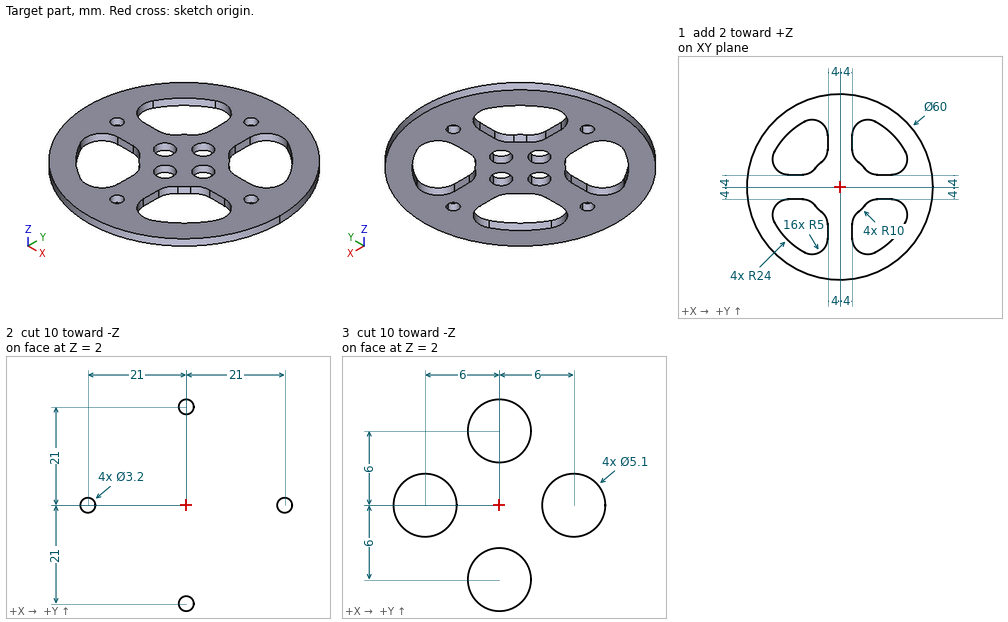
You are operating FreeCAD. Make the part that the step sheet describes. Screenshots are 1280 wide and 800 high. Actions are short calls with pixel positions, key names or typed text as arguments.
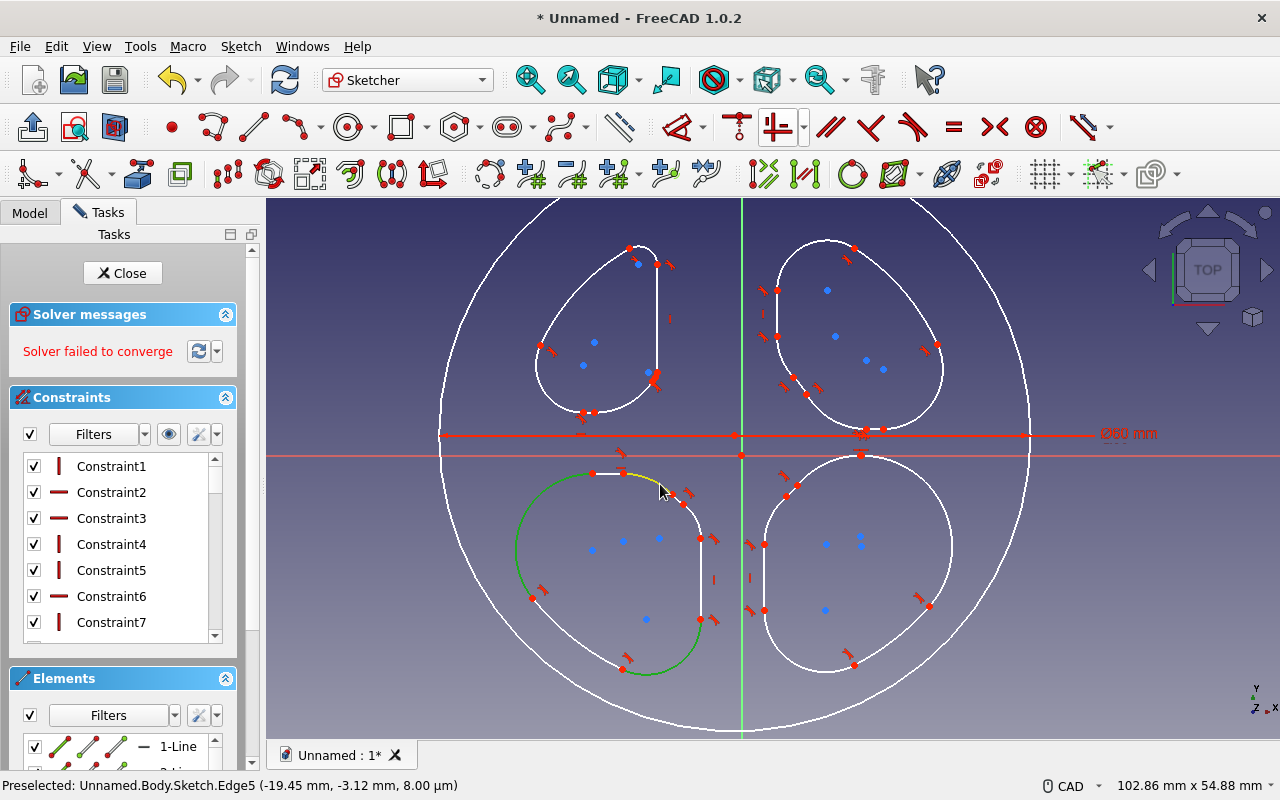
click(660, 484)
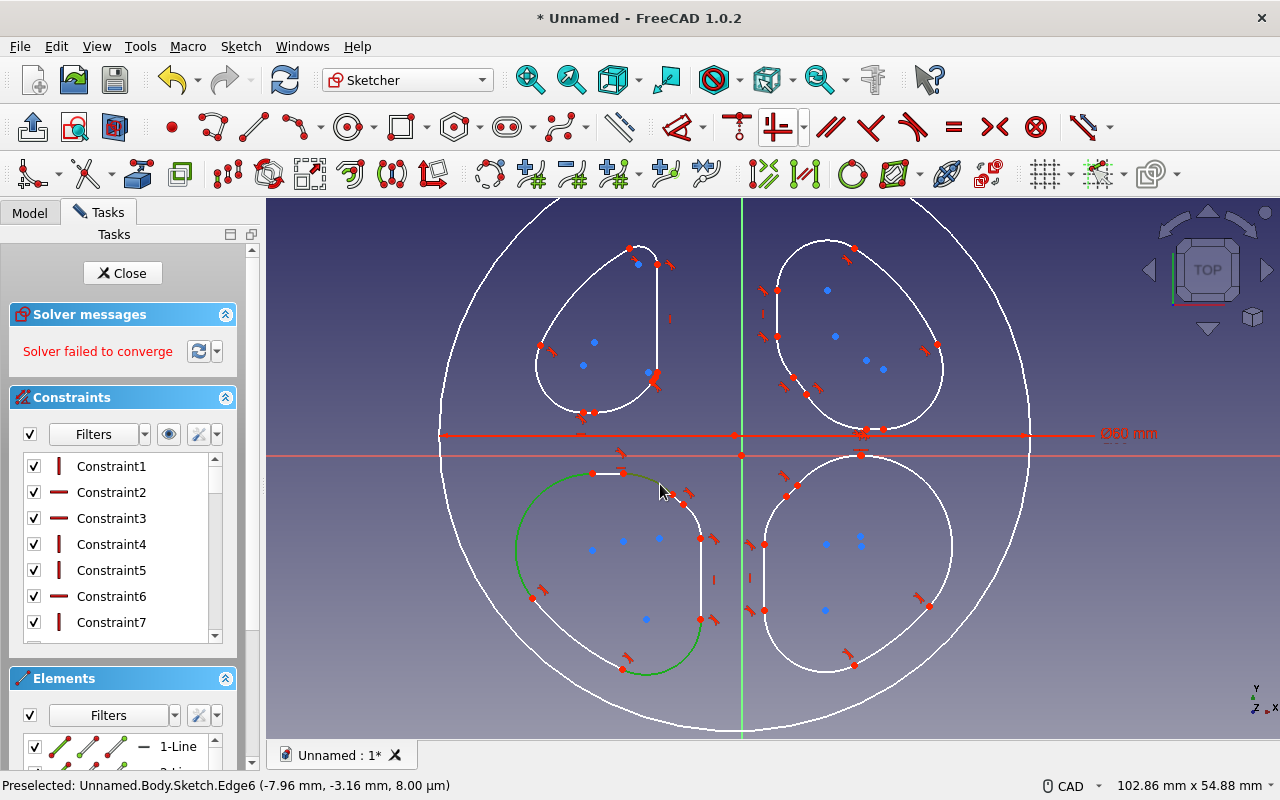
click(699, 527)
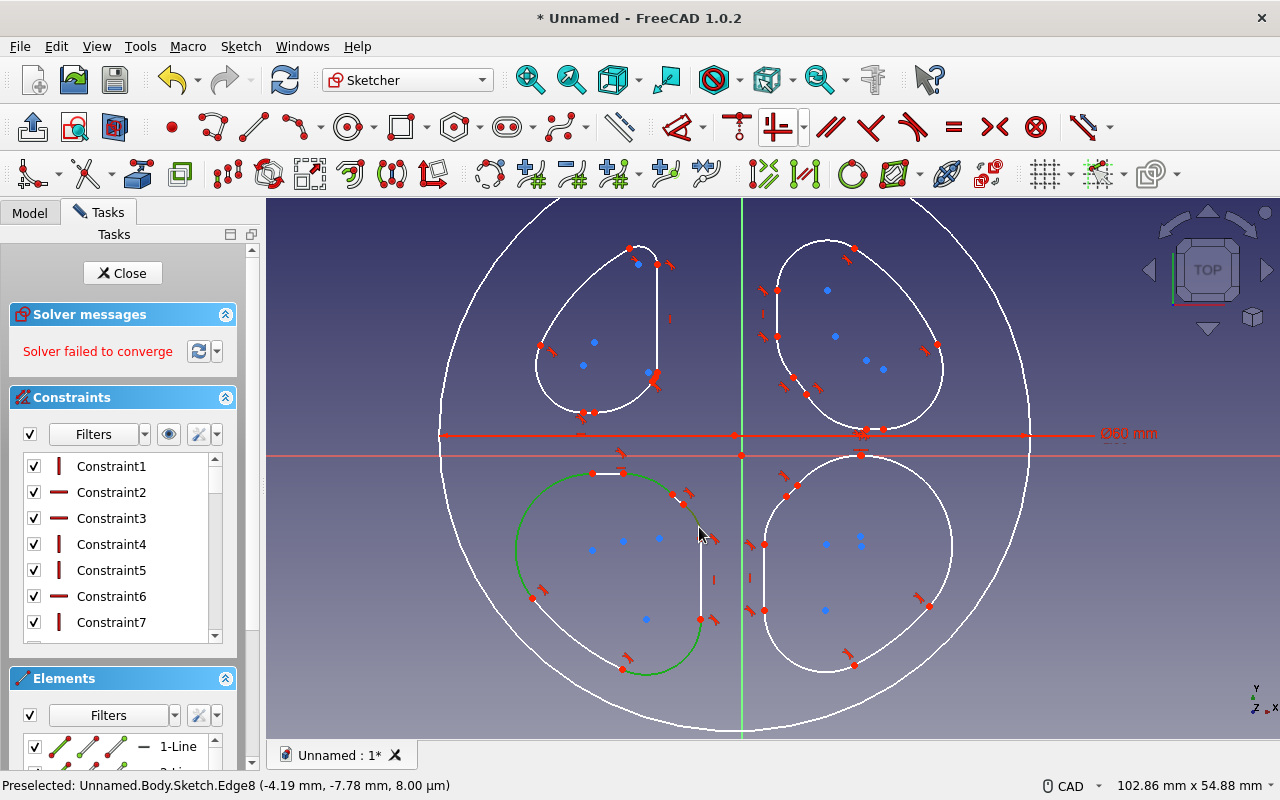
click(952, 549)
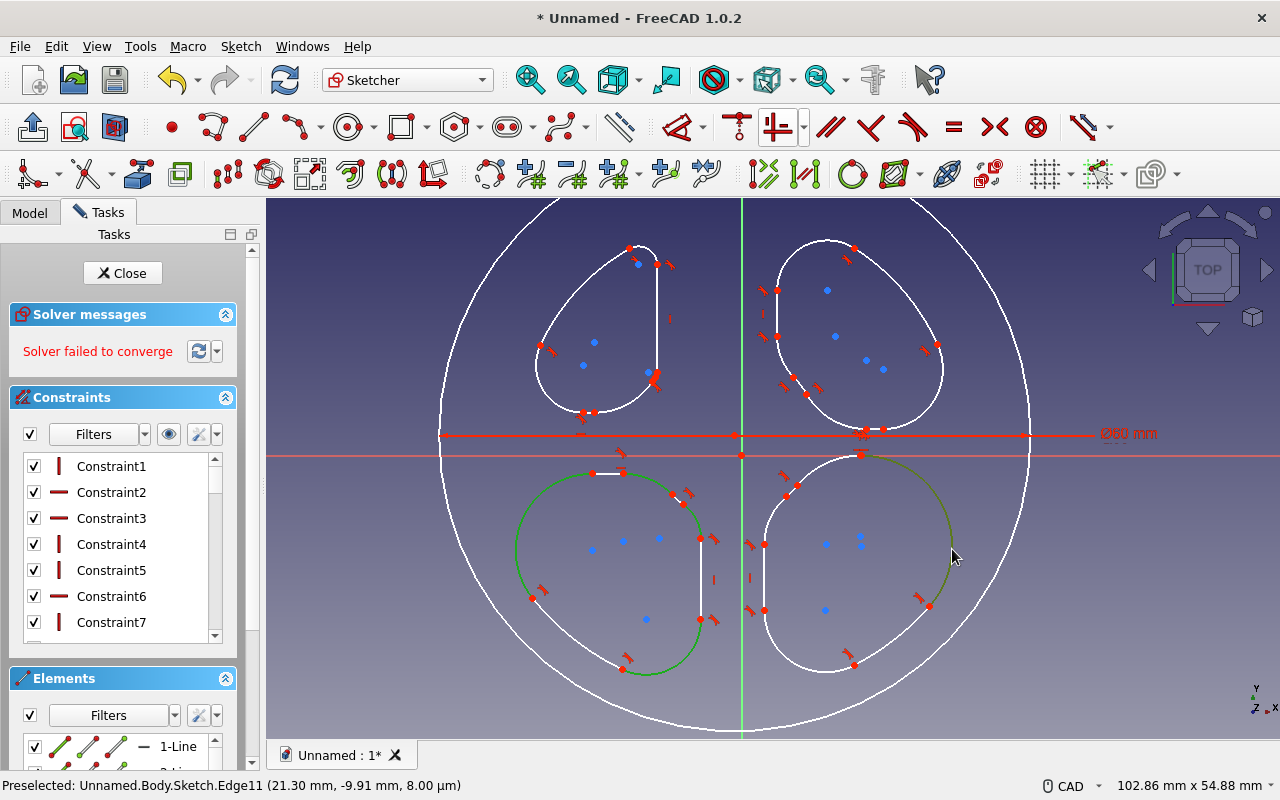
click(776, 646)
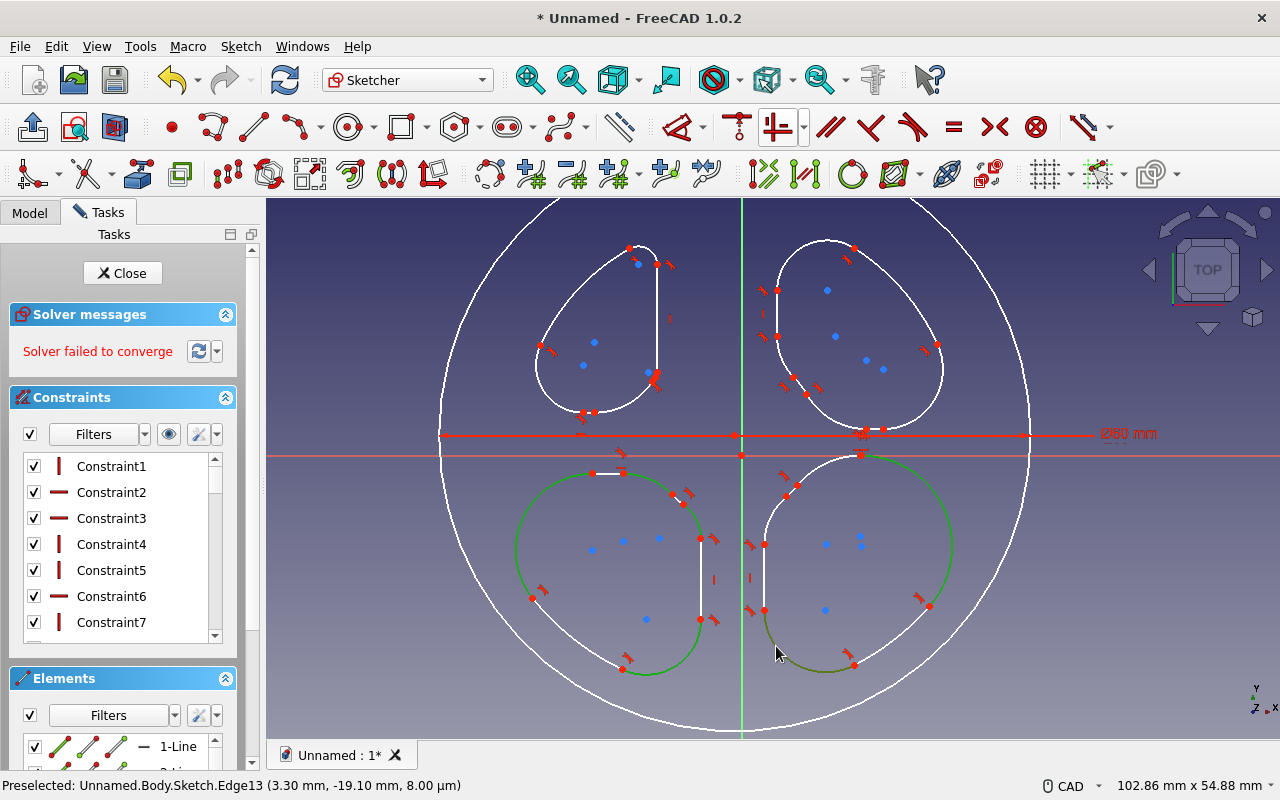
click(776, 509)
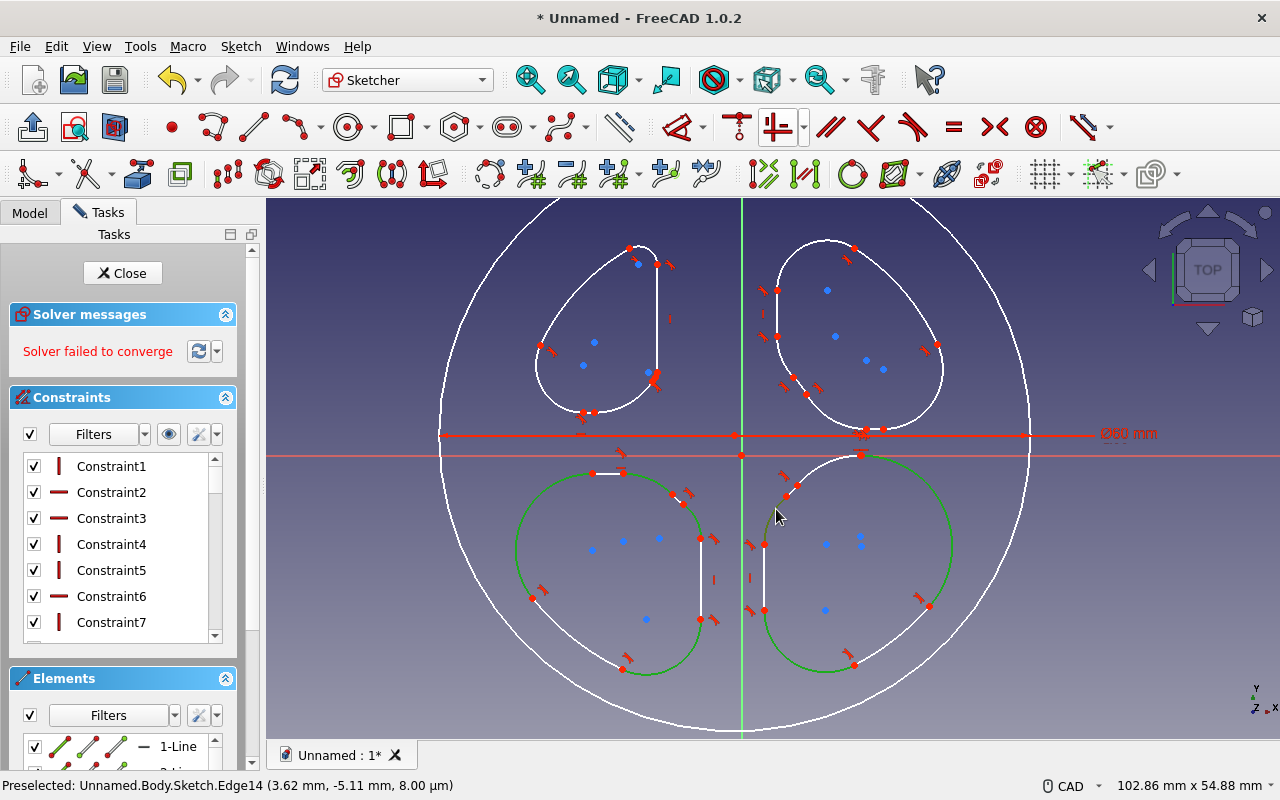
click(839, 459)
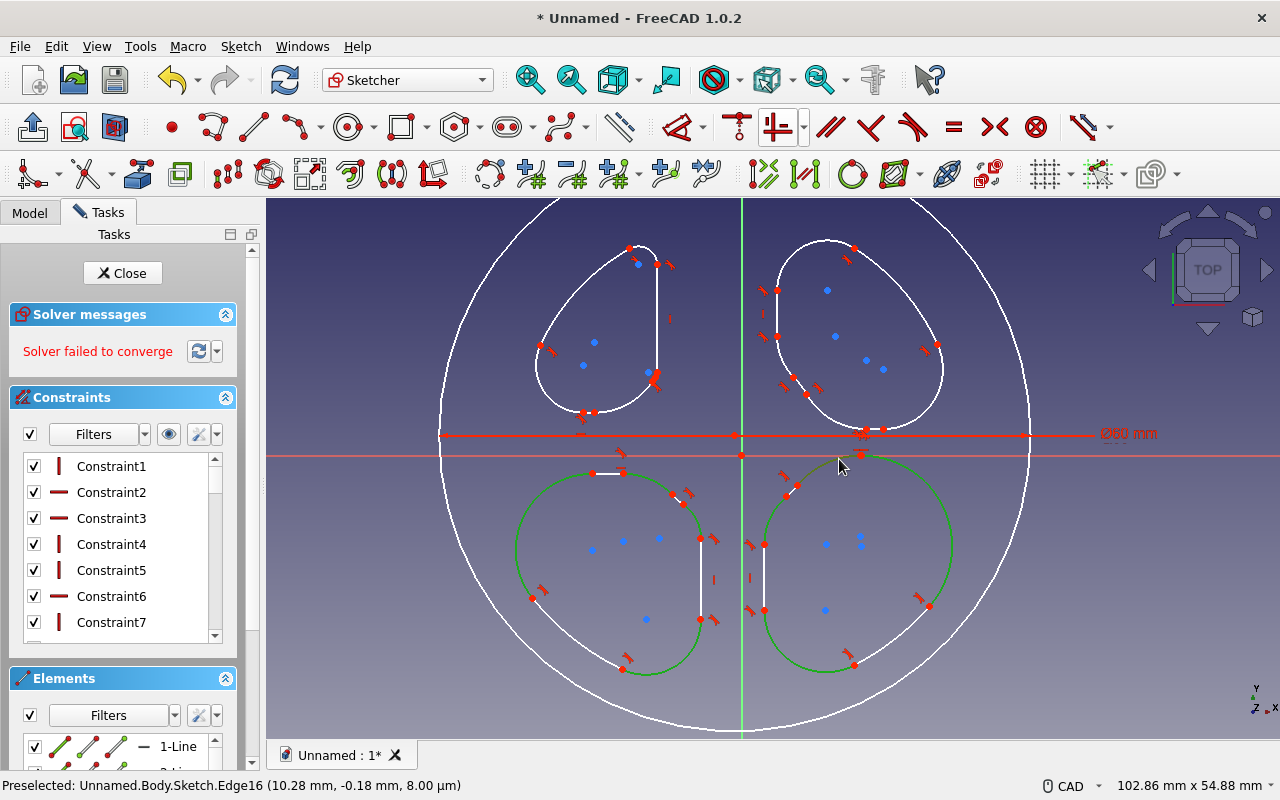
scroll(657, 375, up, 9)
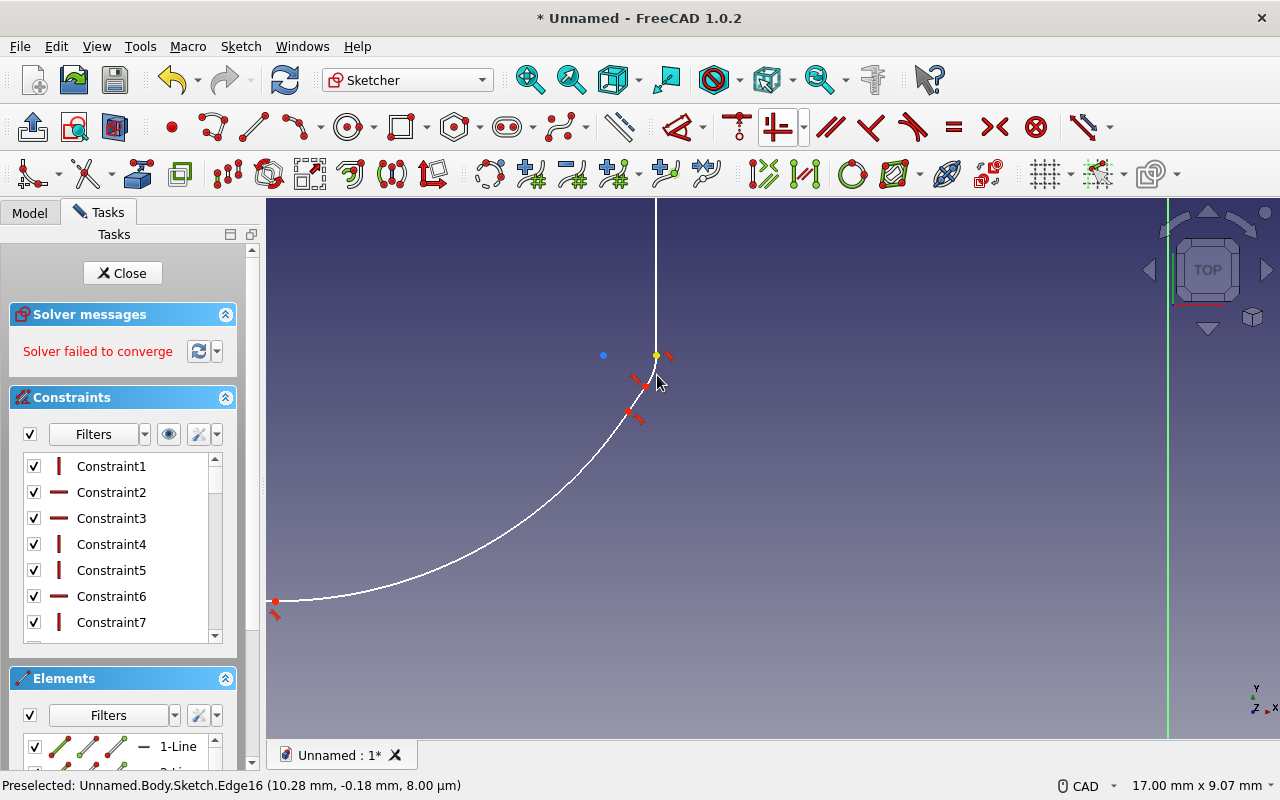
click(654, 372)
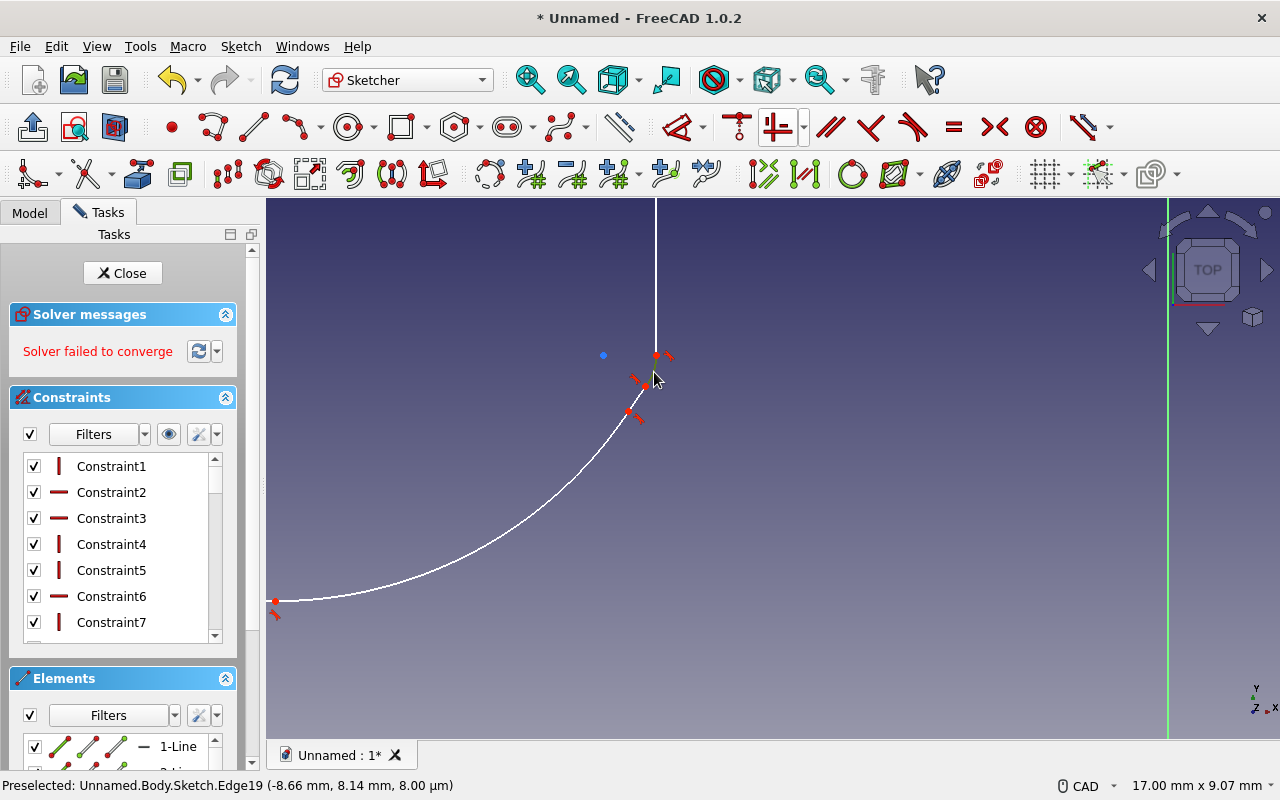
scroll(658, 429, down, 12)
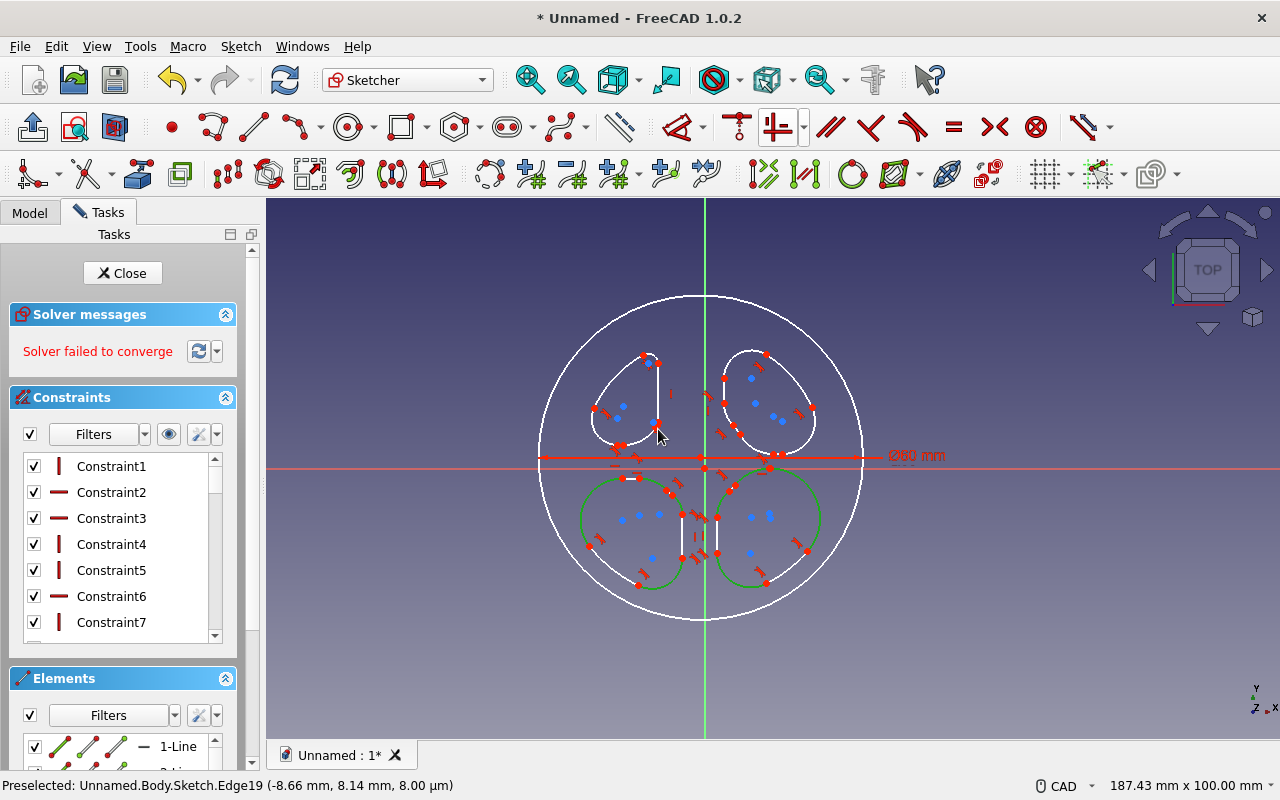
click(635, 443)